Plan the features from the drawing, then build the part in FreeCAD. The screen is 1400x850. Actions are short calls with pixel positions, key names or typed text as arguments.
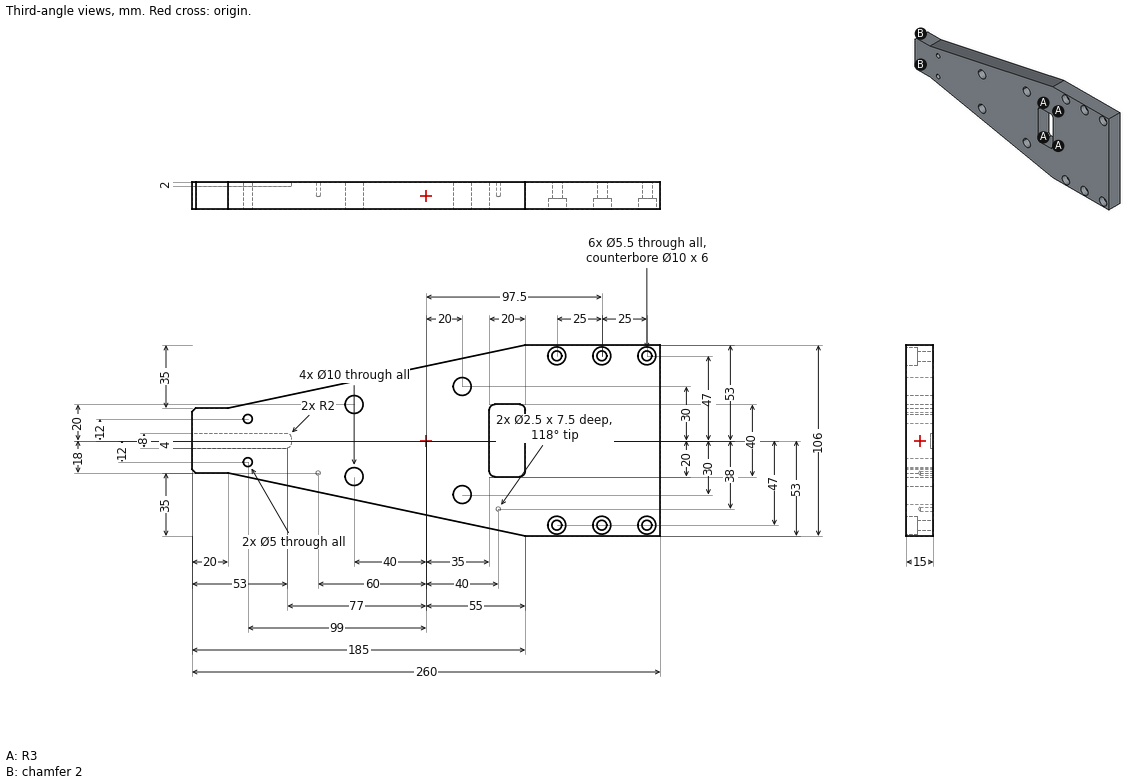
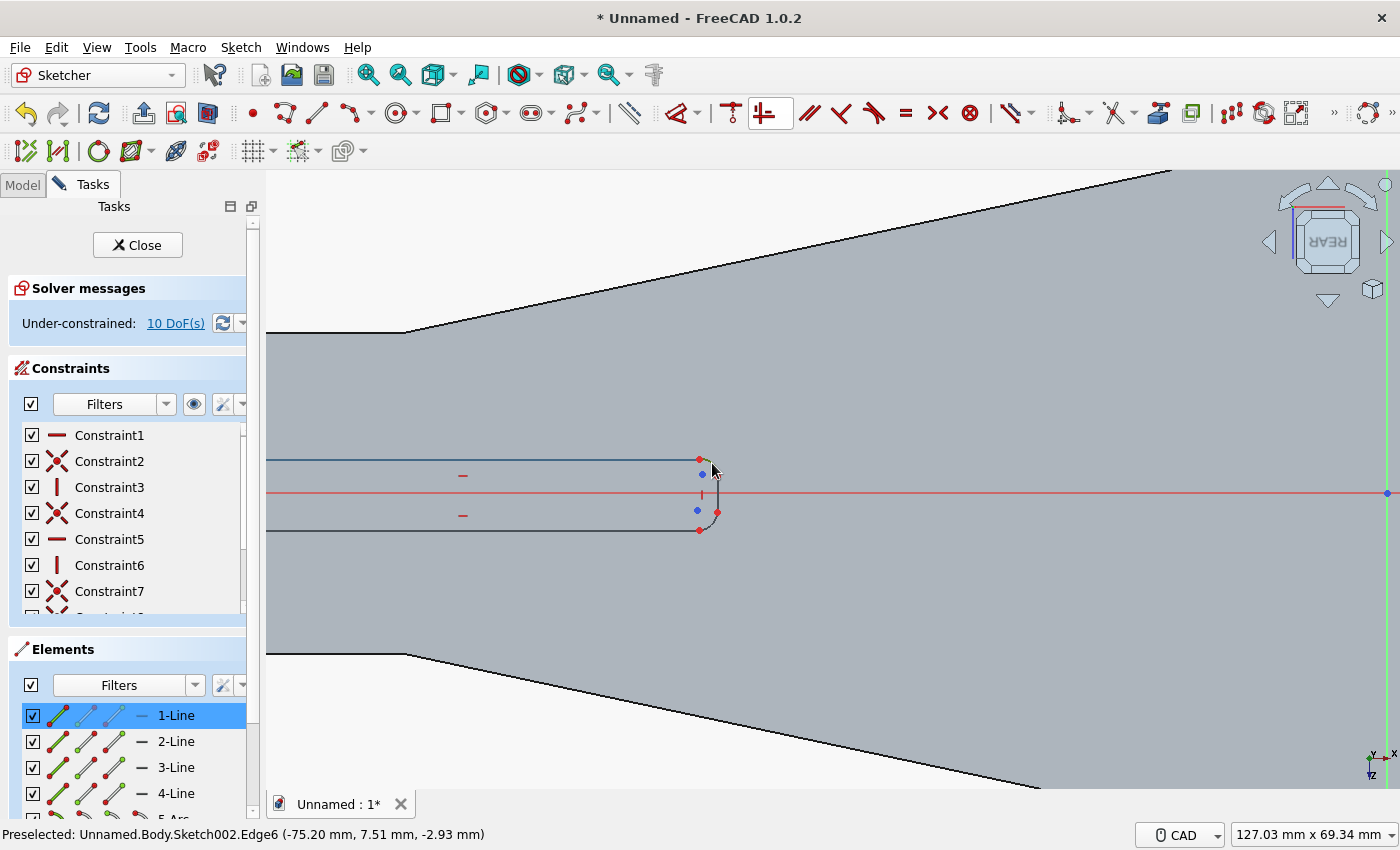
click(874, 114)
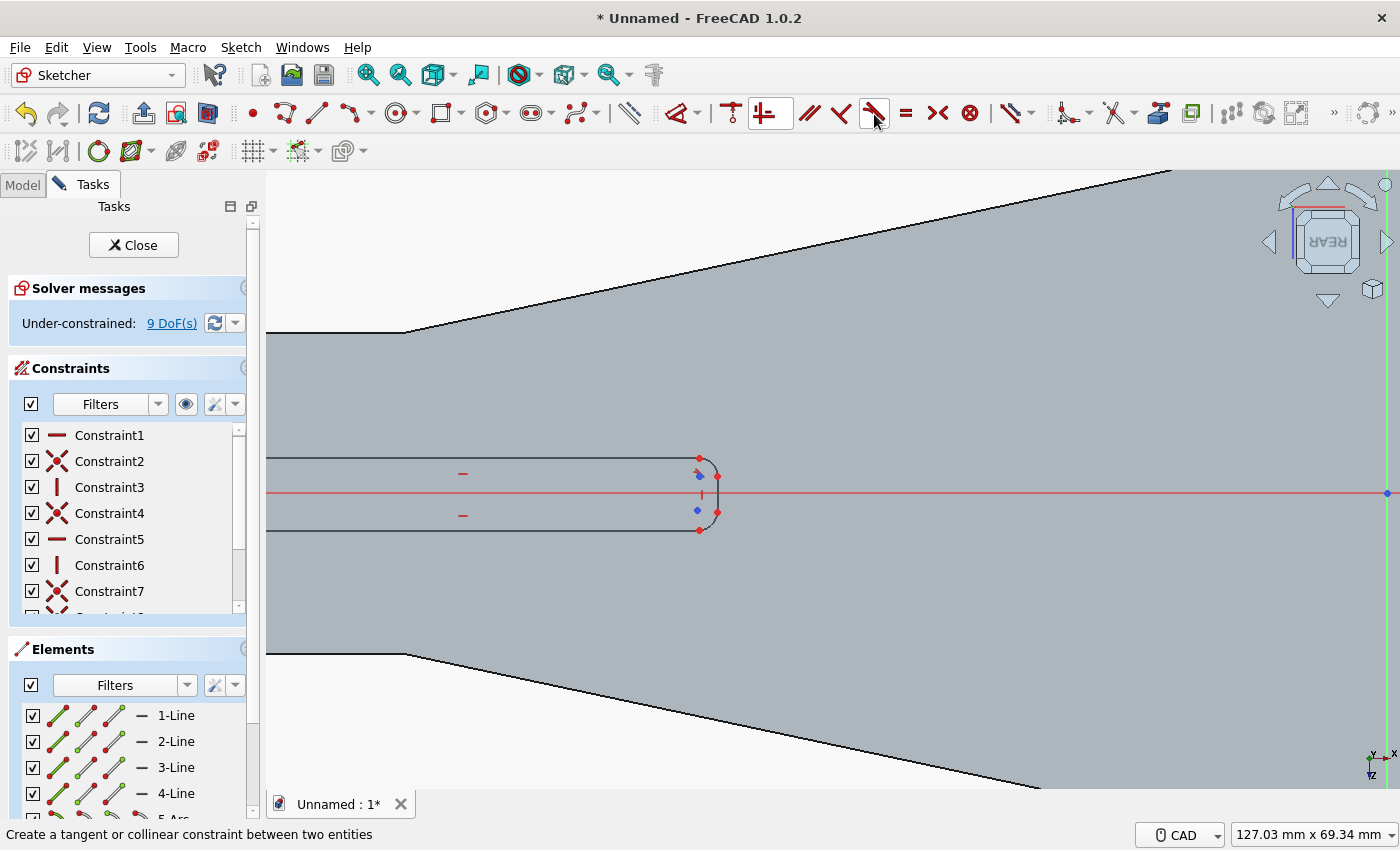
click(369, 531)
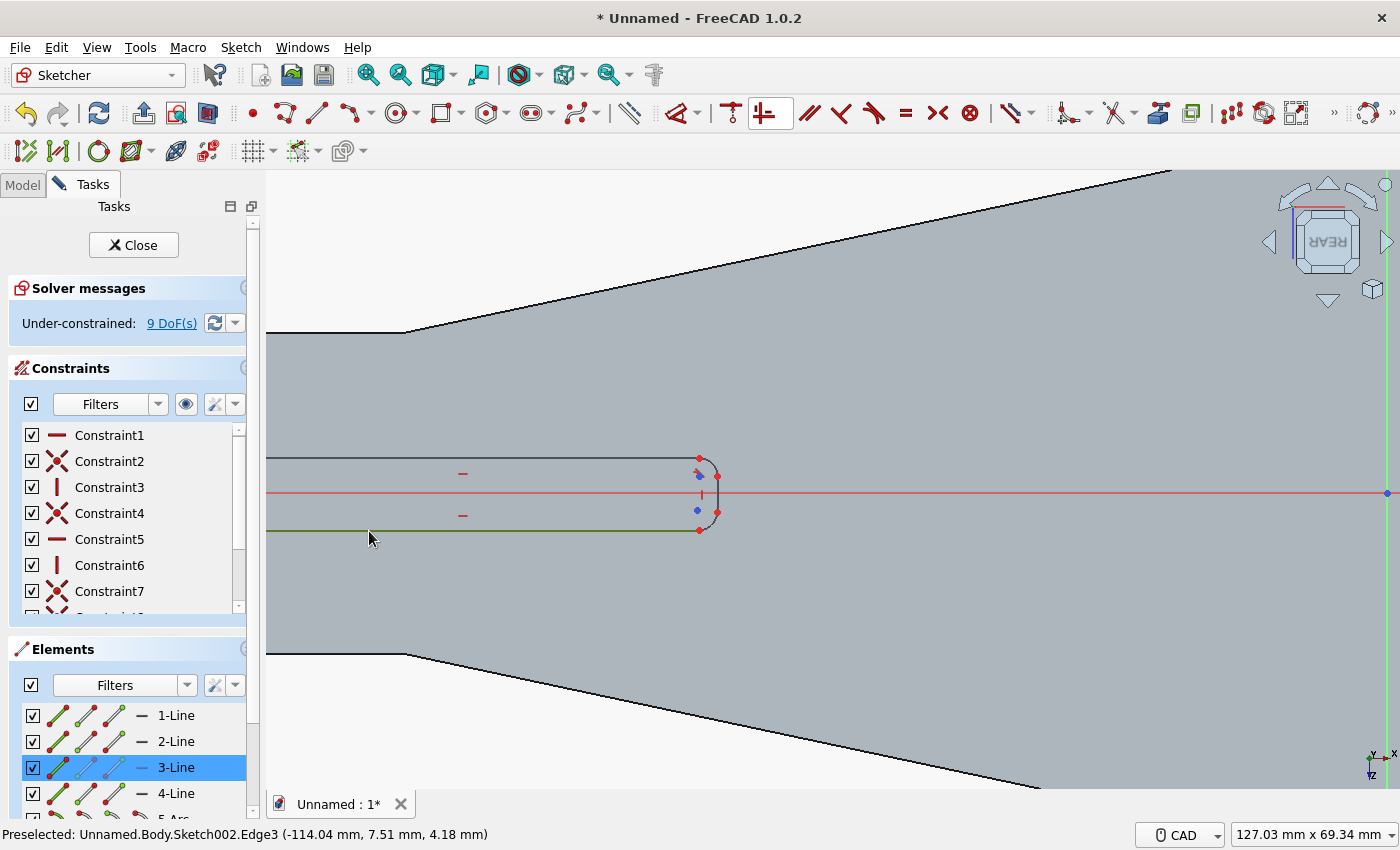
click(712, 525)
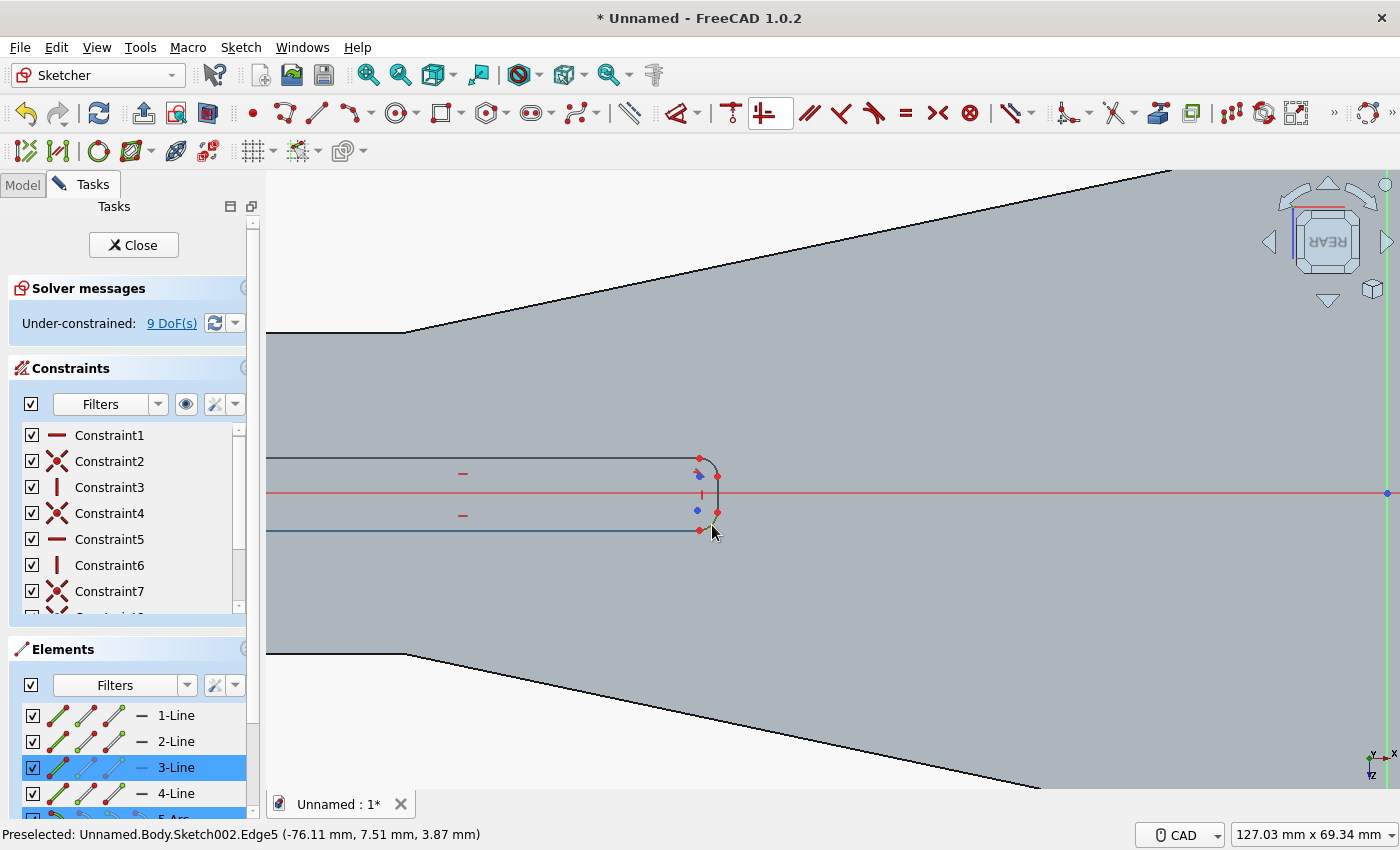
key(t)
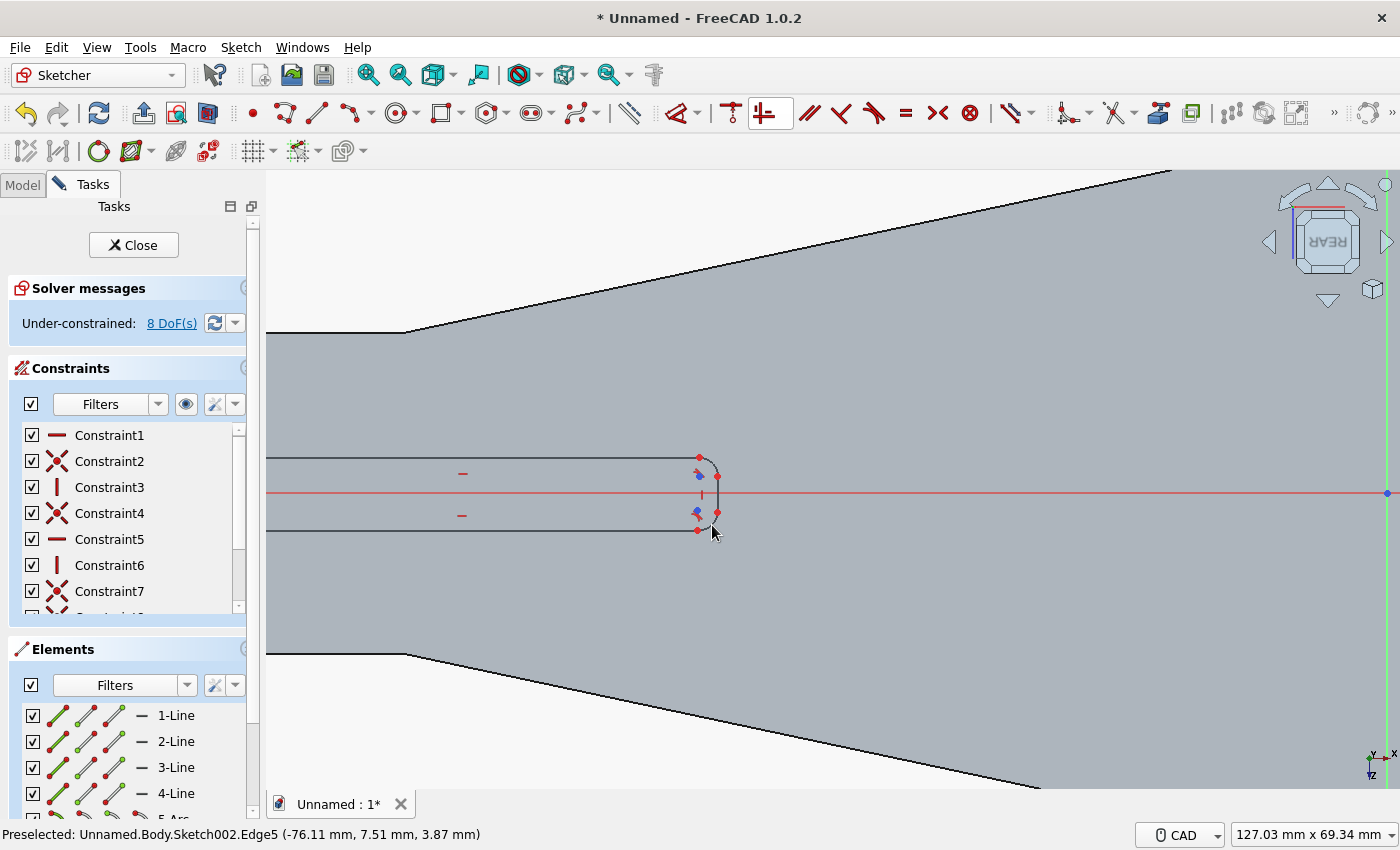
click(718, 491)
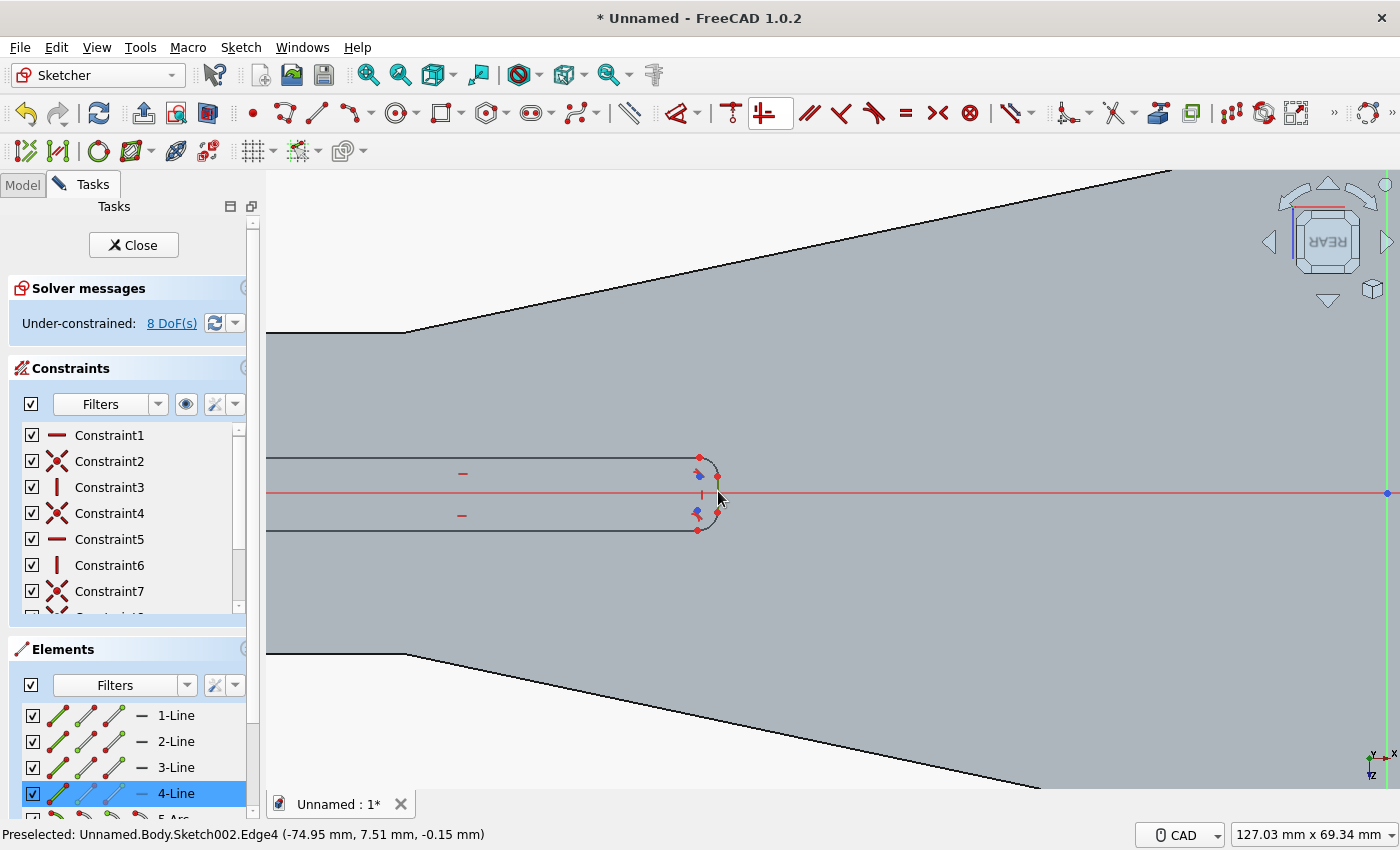
click(711, 525)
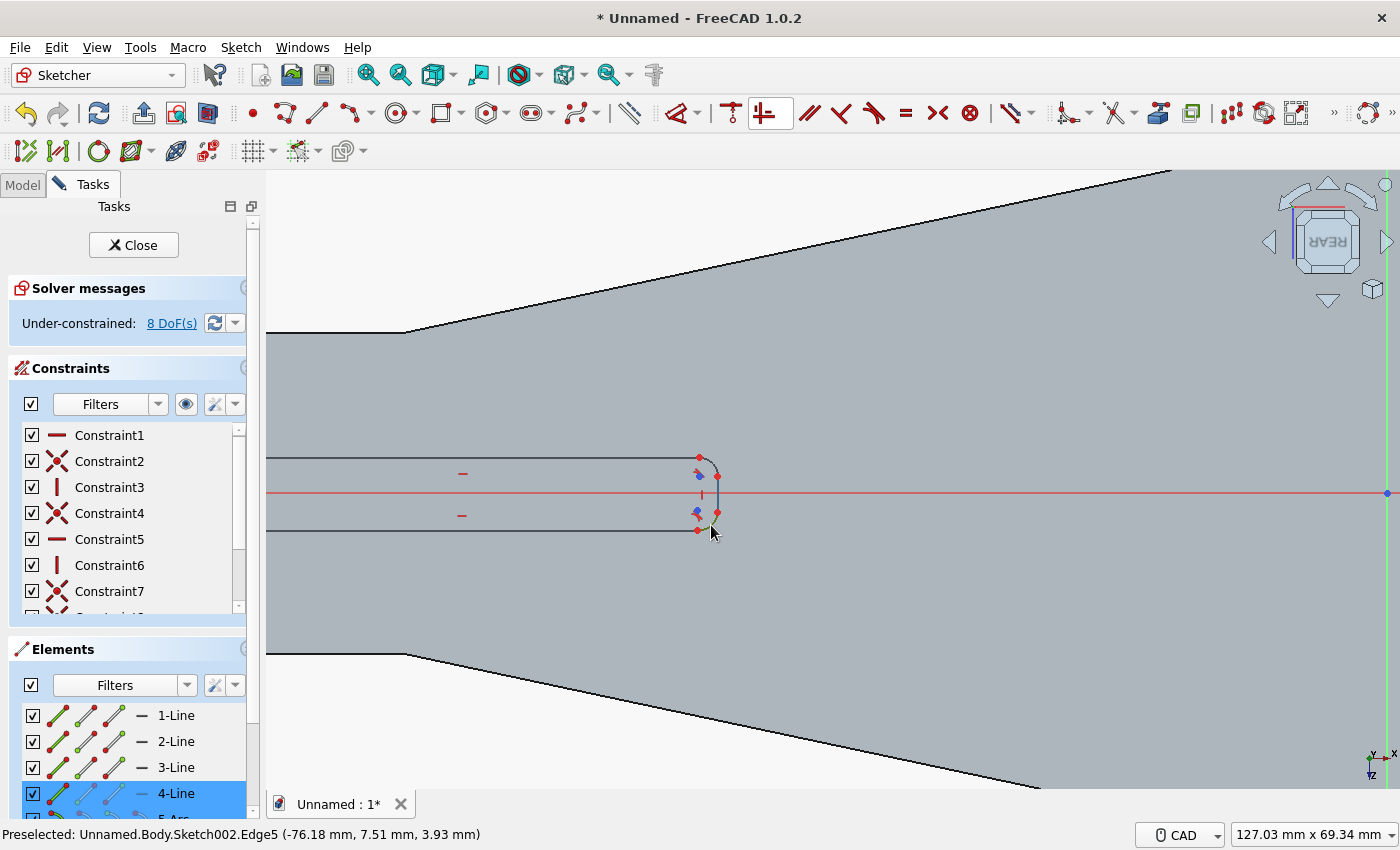
key(t)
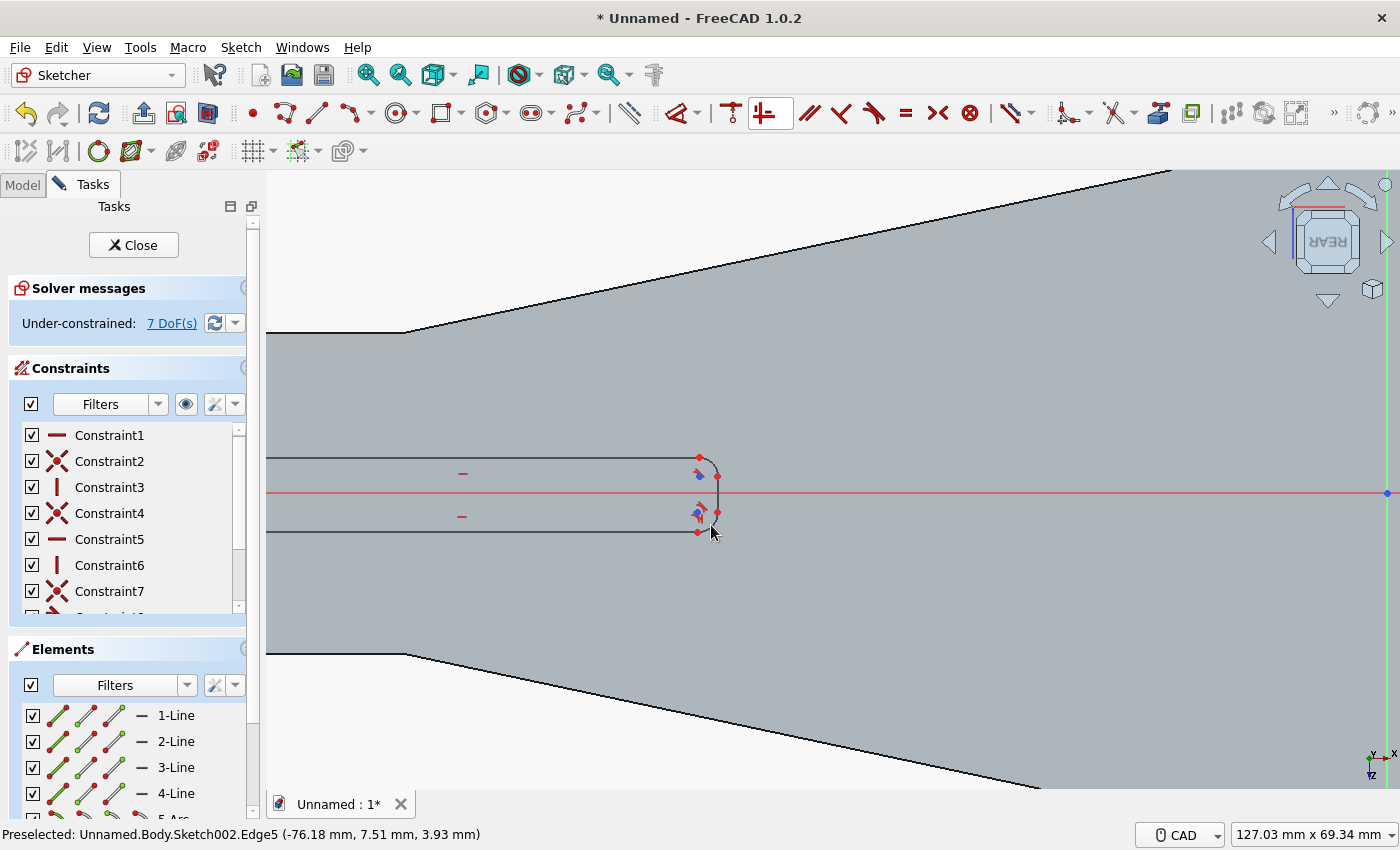
click(718, 490)